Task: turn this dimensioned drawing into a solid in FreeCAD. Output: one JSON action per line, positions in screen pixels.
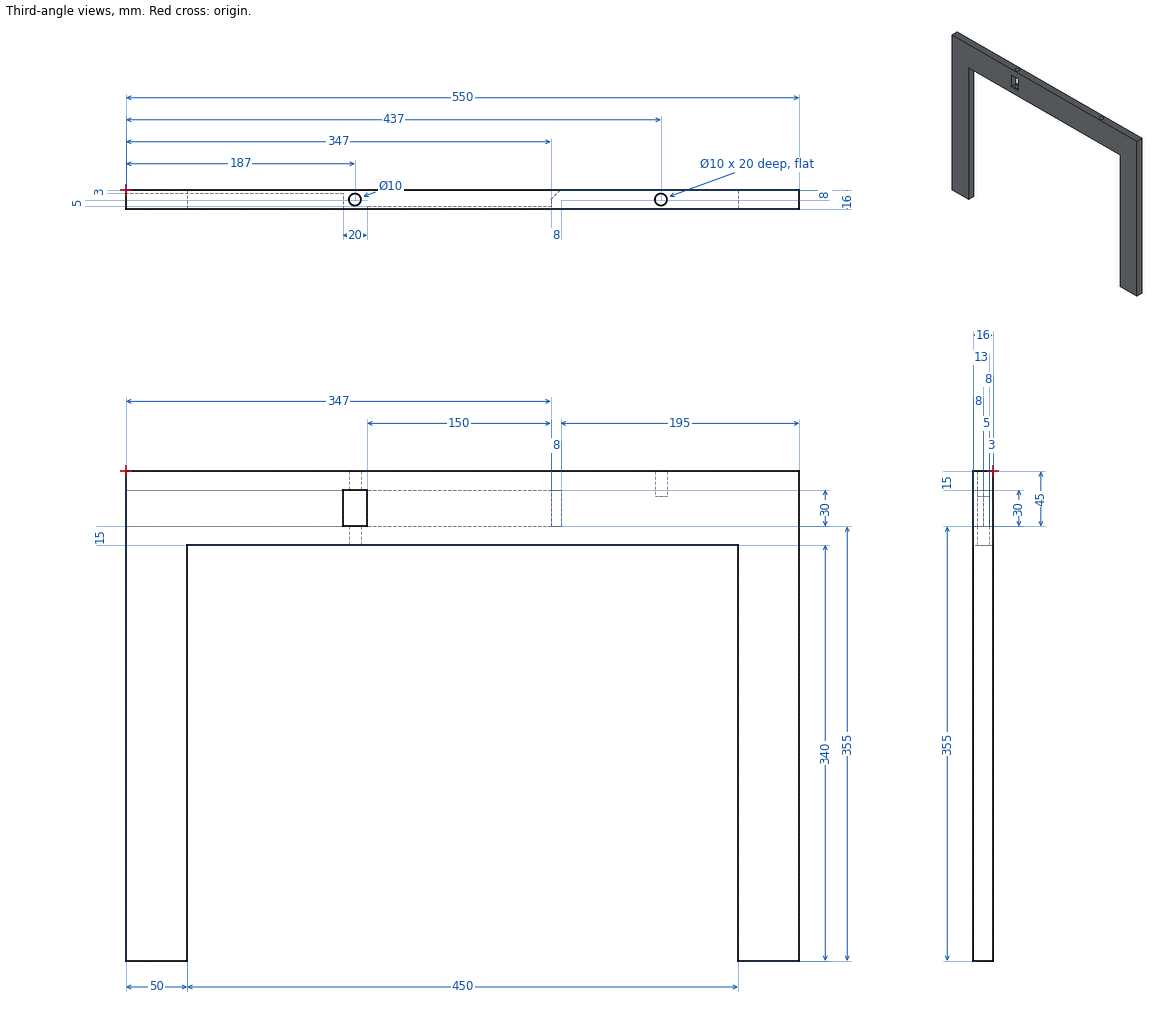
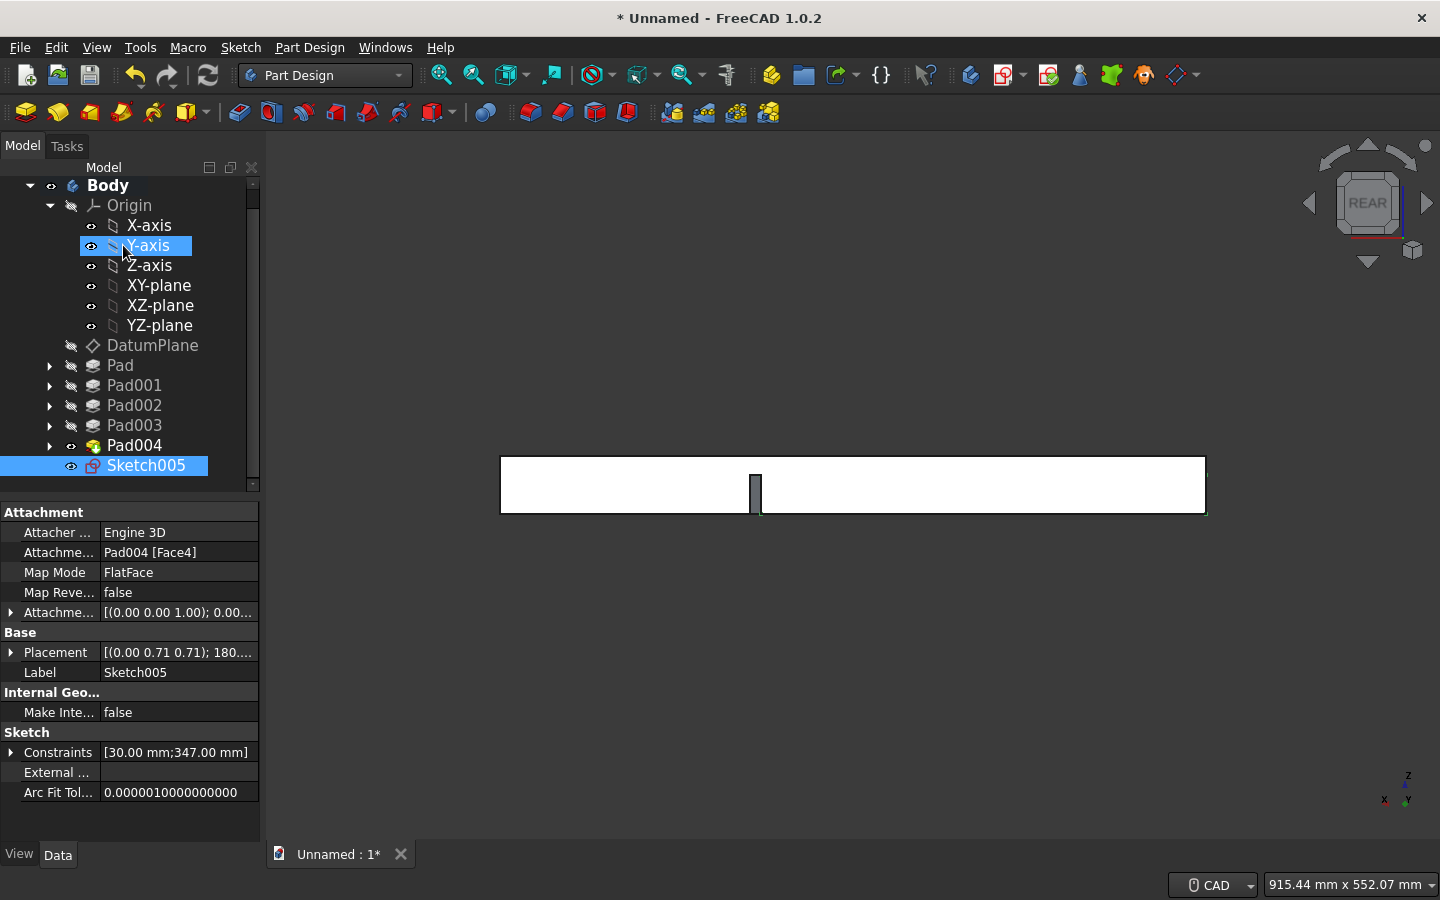
{"action": "left_click", "coordinate": [240, 112]}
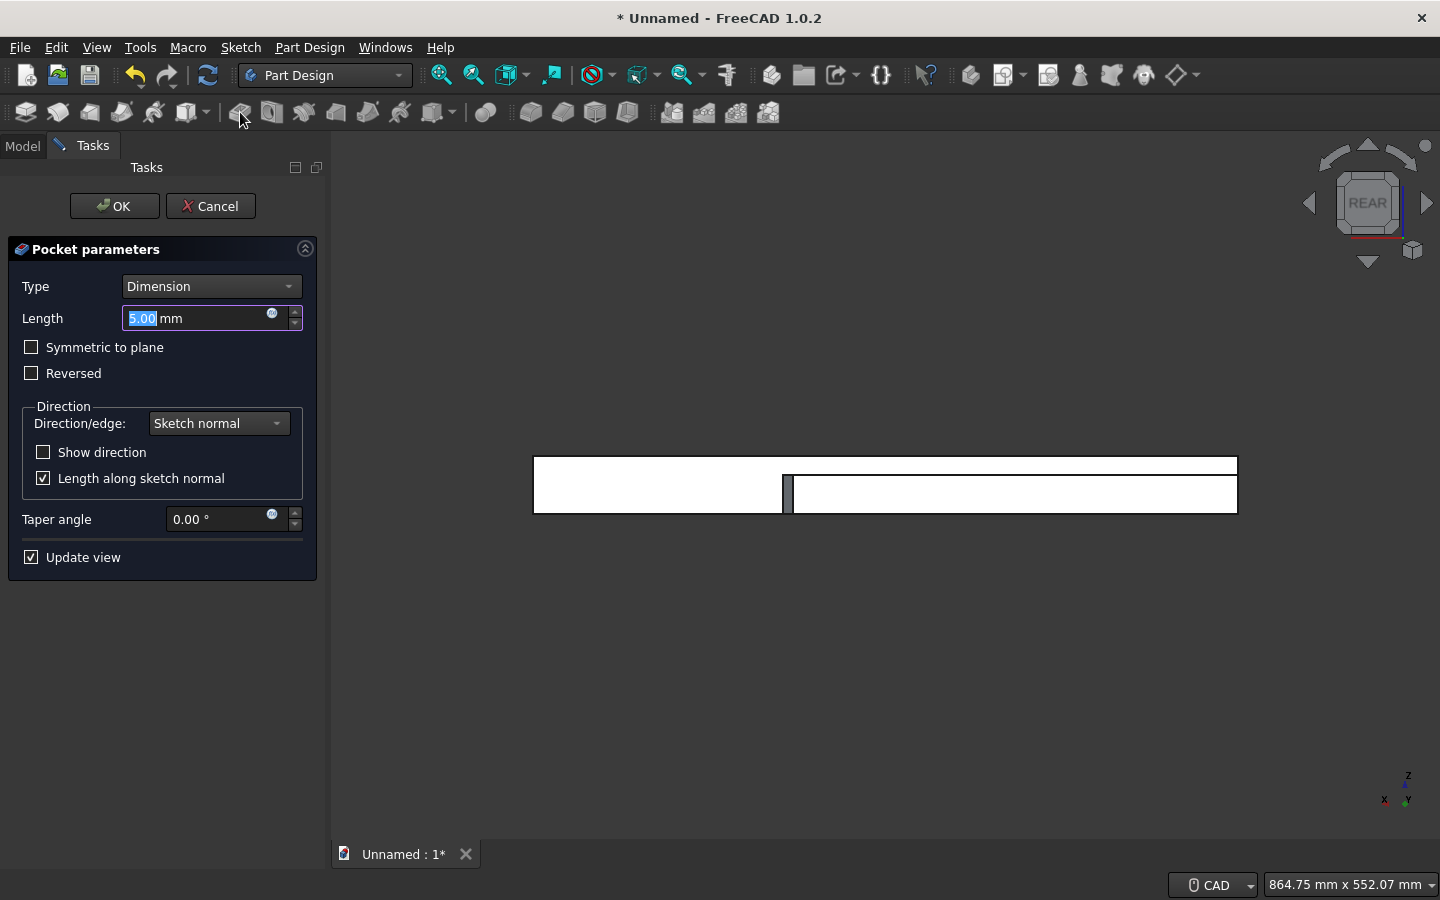
{"action": "type", "text": "3"}
{"action": "key", "text": "Tab"}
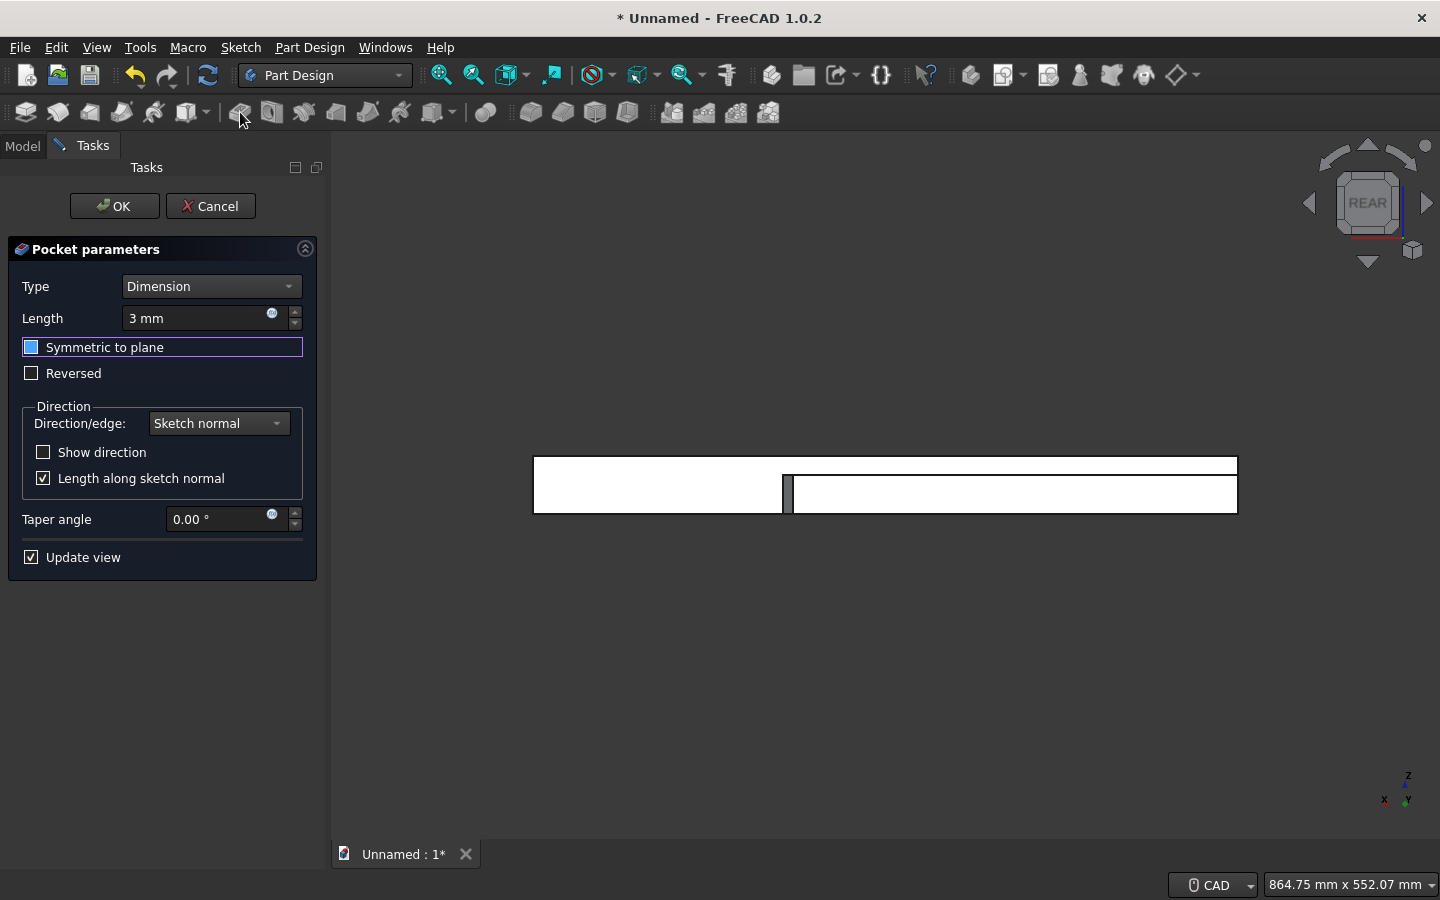
{"action": "left_click", "coordinate": [115, 206]}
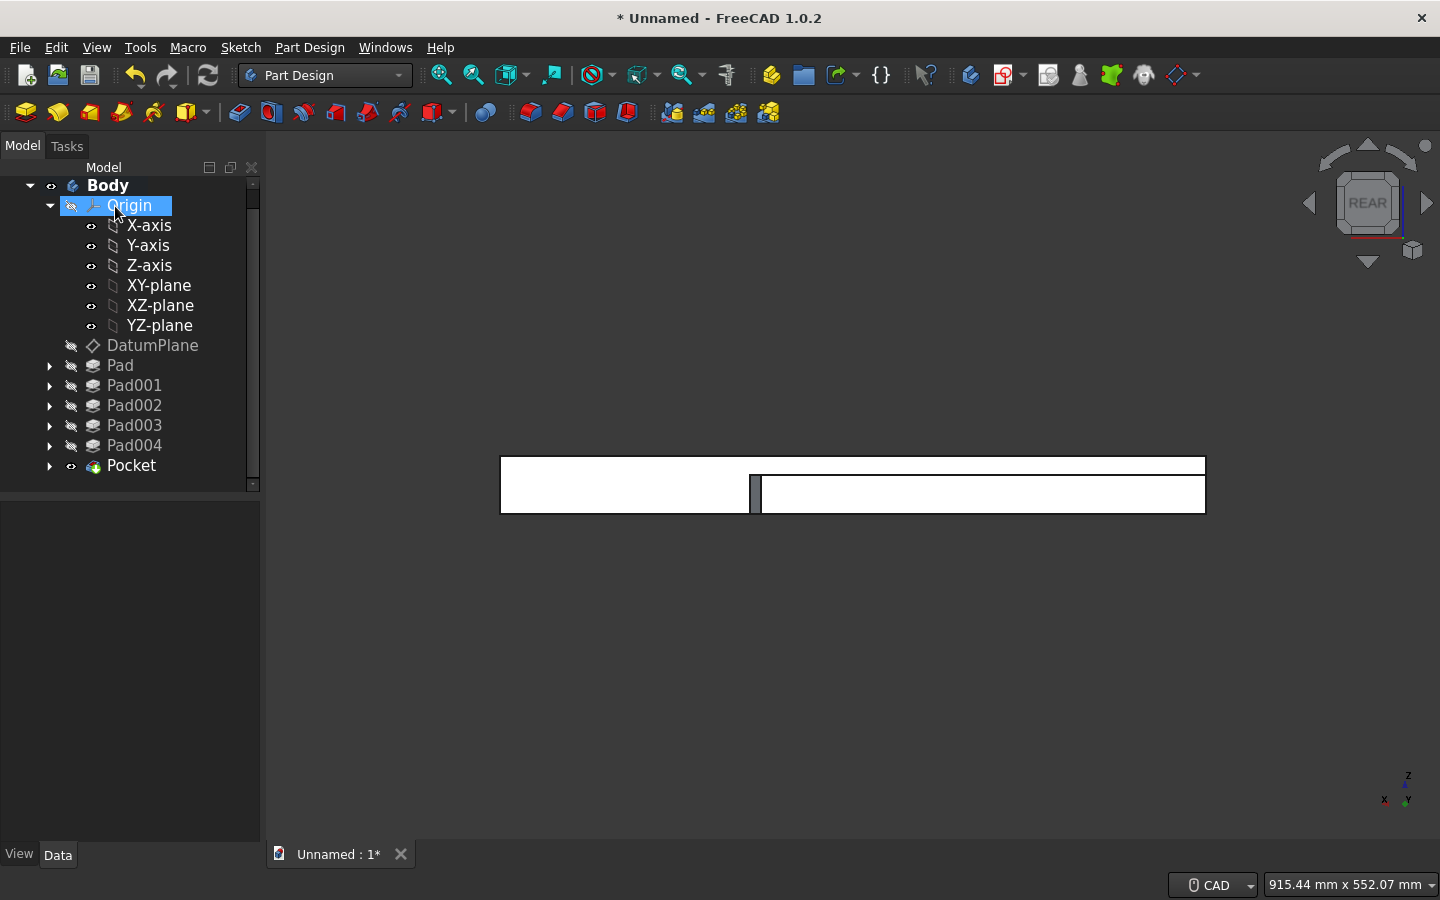
{"action": "left_click", "coordinate": [136, 326]}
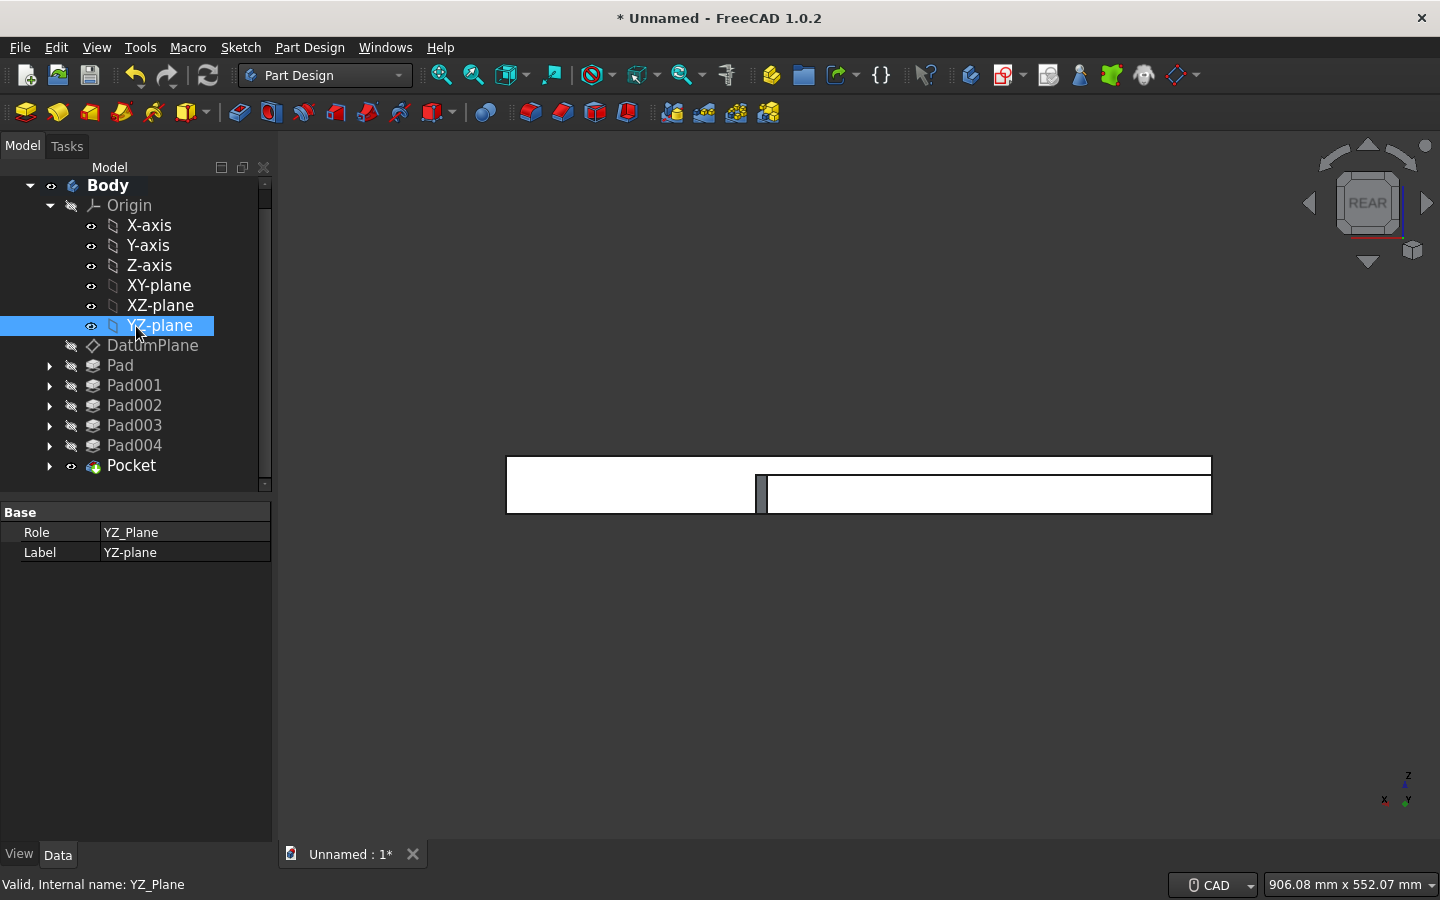
{"action": "left_click", "coordinate": [1176, 76]}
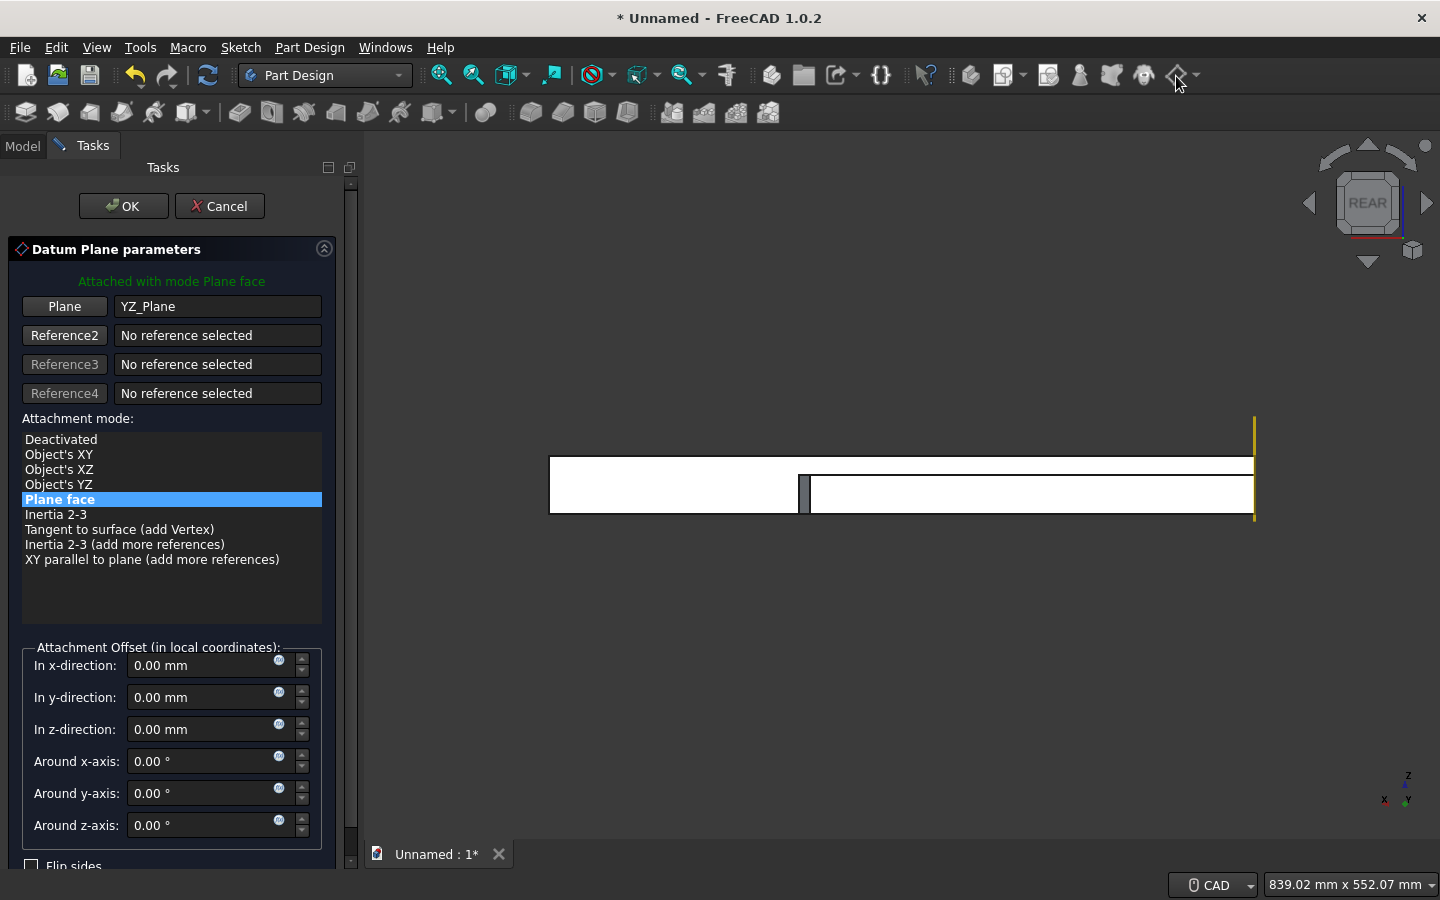
{"action": "triple_click", "coordinate": [210, 729]}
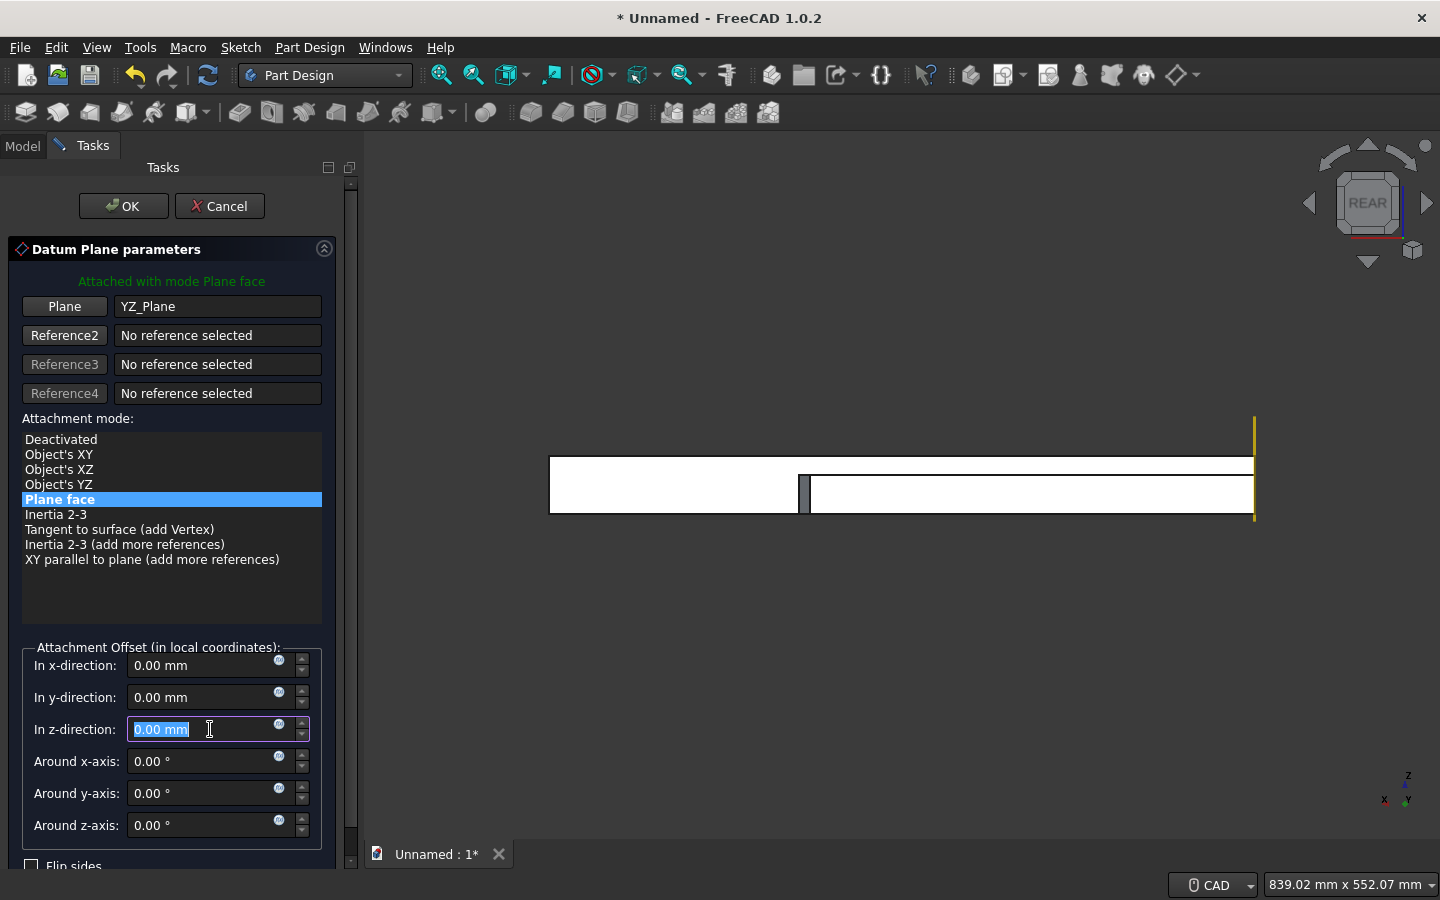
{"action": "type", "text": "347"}
{"action": "key", "text": "Tab"}